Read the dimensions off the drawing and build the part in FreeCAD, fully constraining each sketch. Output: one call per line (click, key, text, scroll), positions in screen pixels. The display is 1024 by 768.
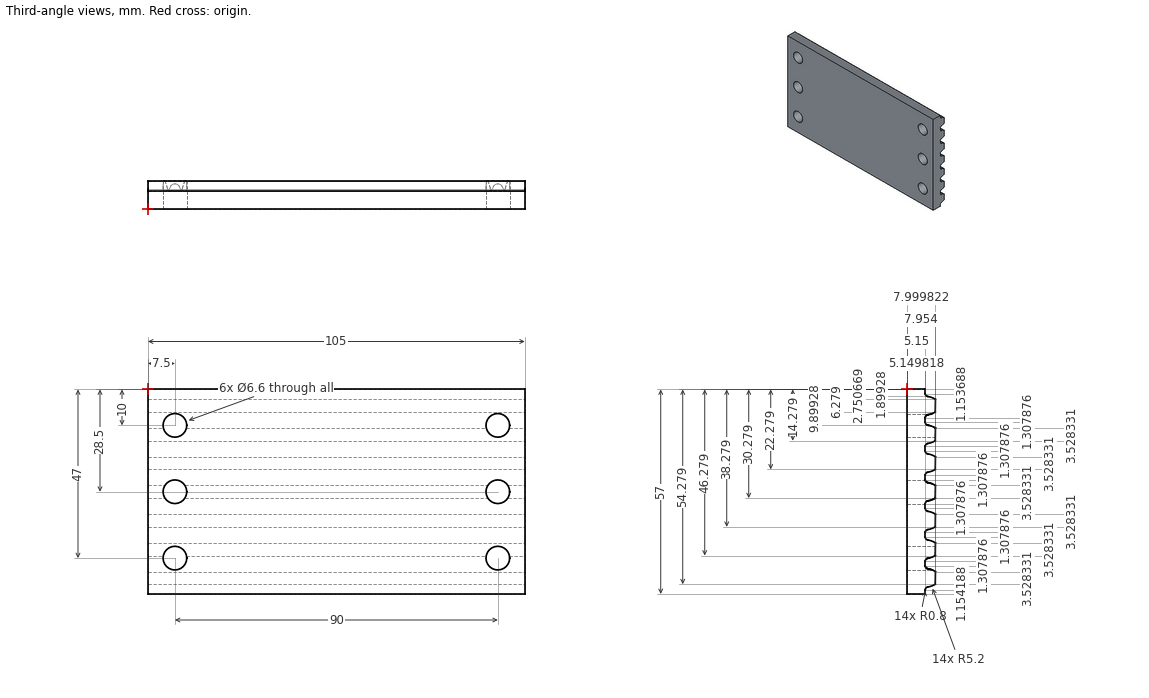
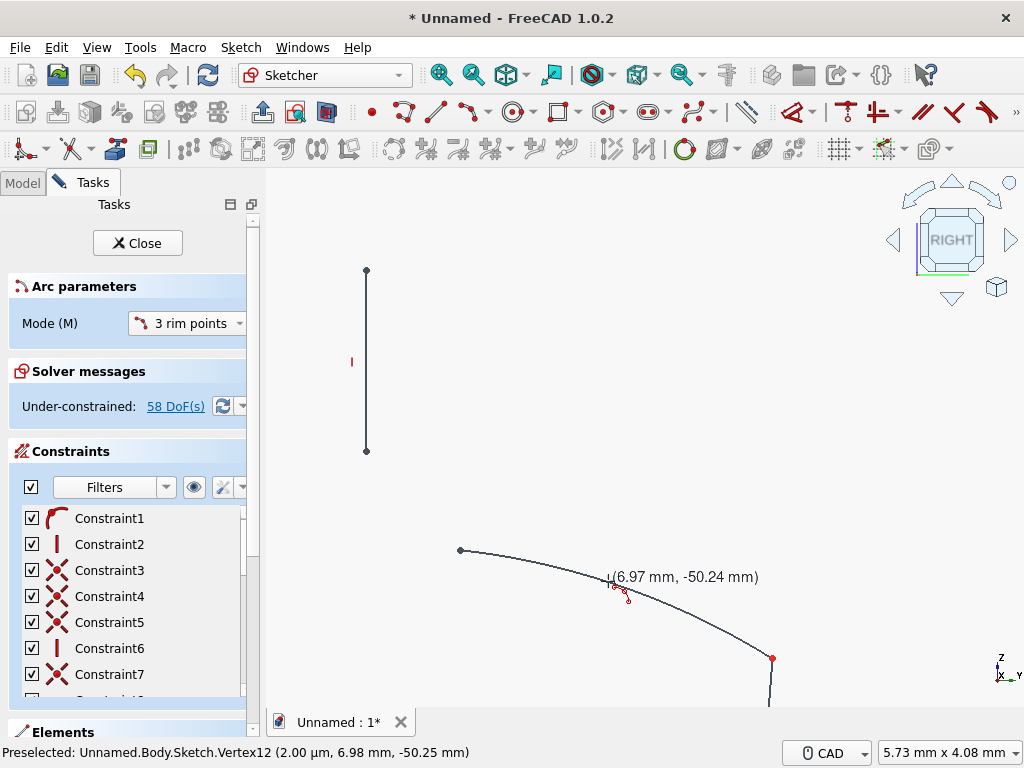
scroll(595, 581, down, 15)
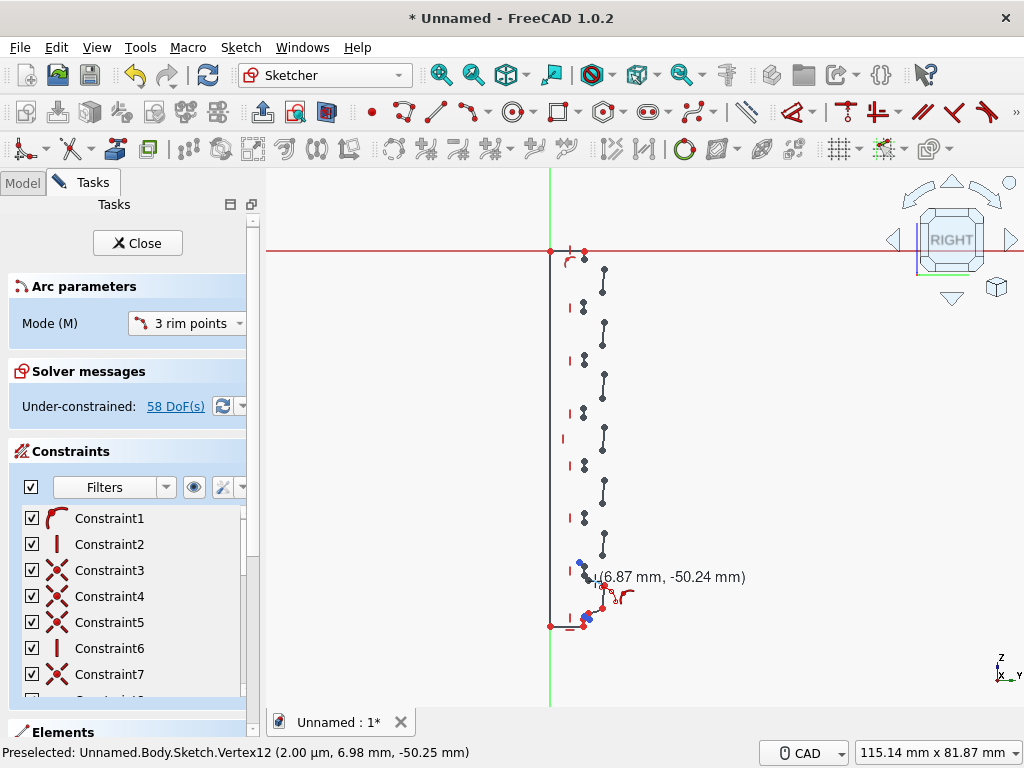
scroll(589, 580, up, 7)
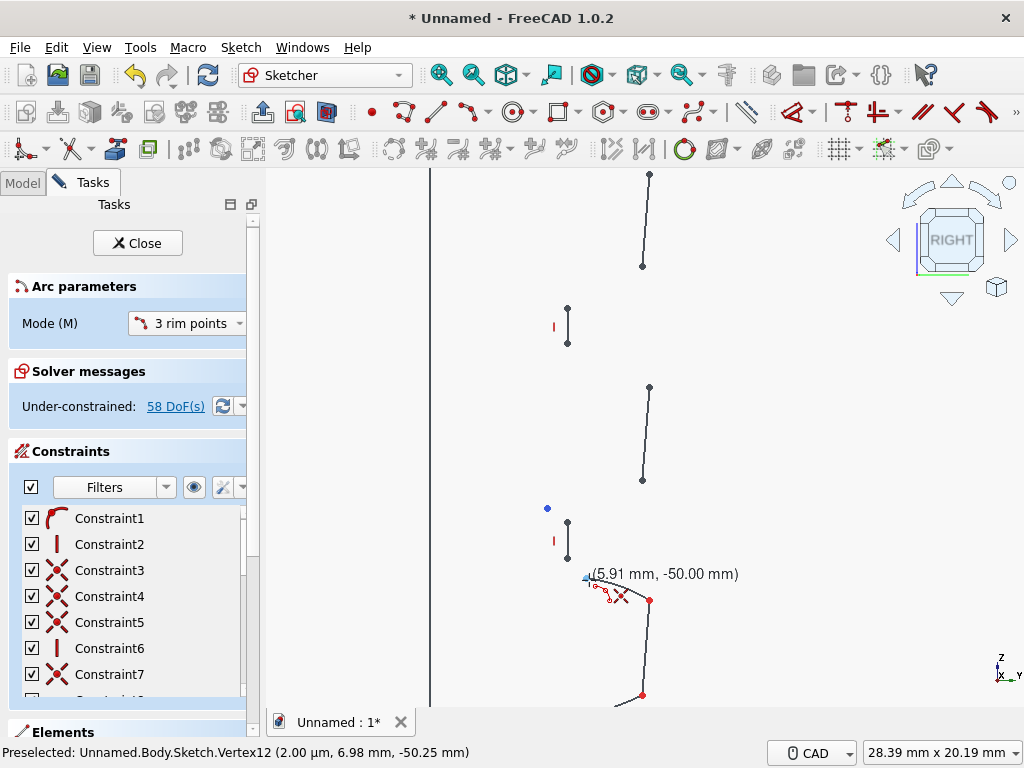
click(587, 578)
click(568, 558)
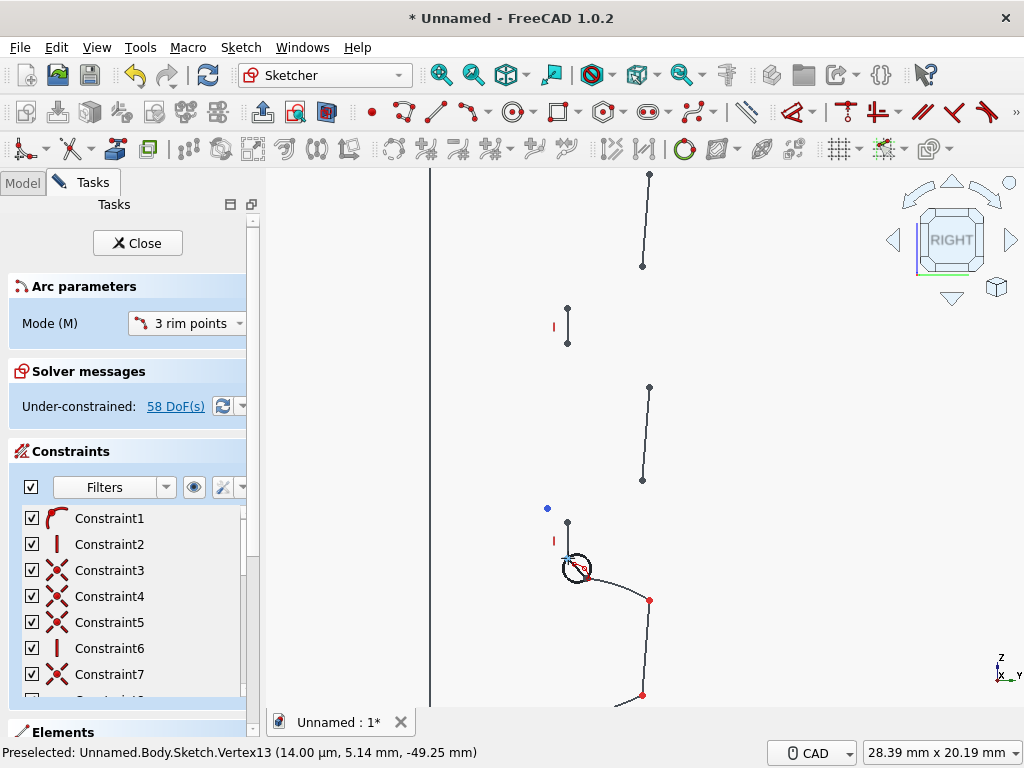
scroll(573, 570, up, 6)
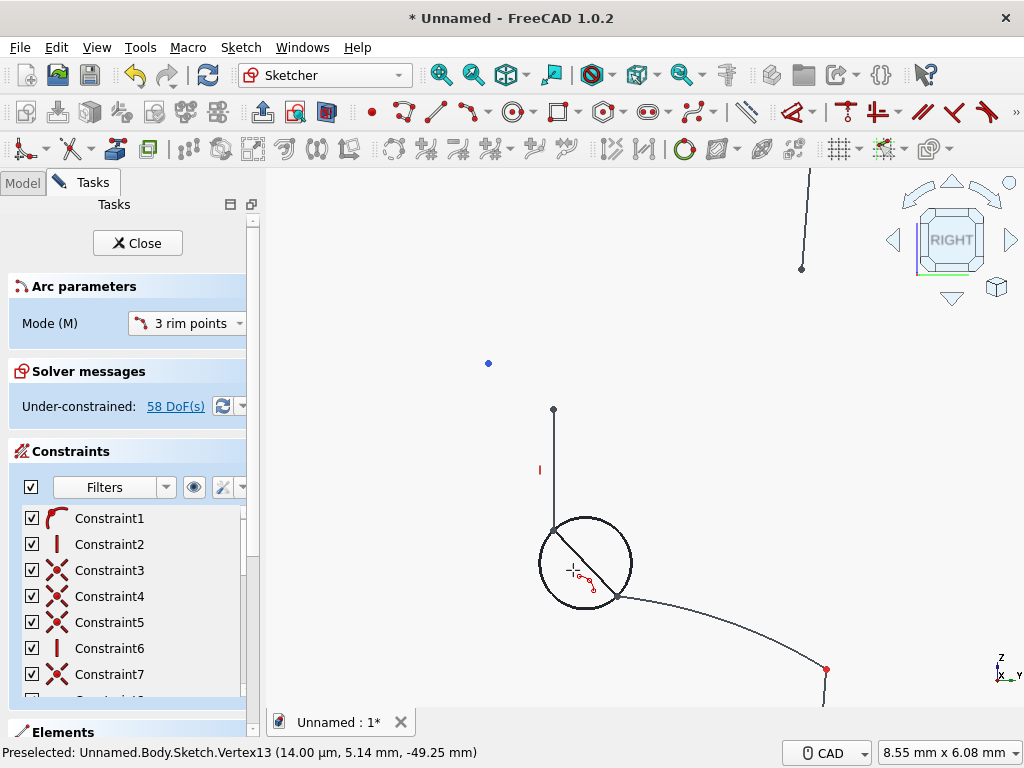
click(572, 568)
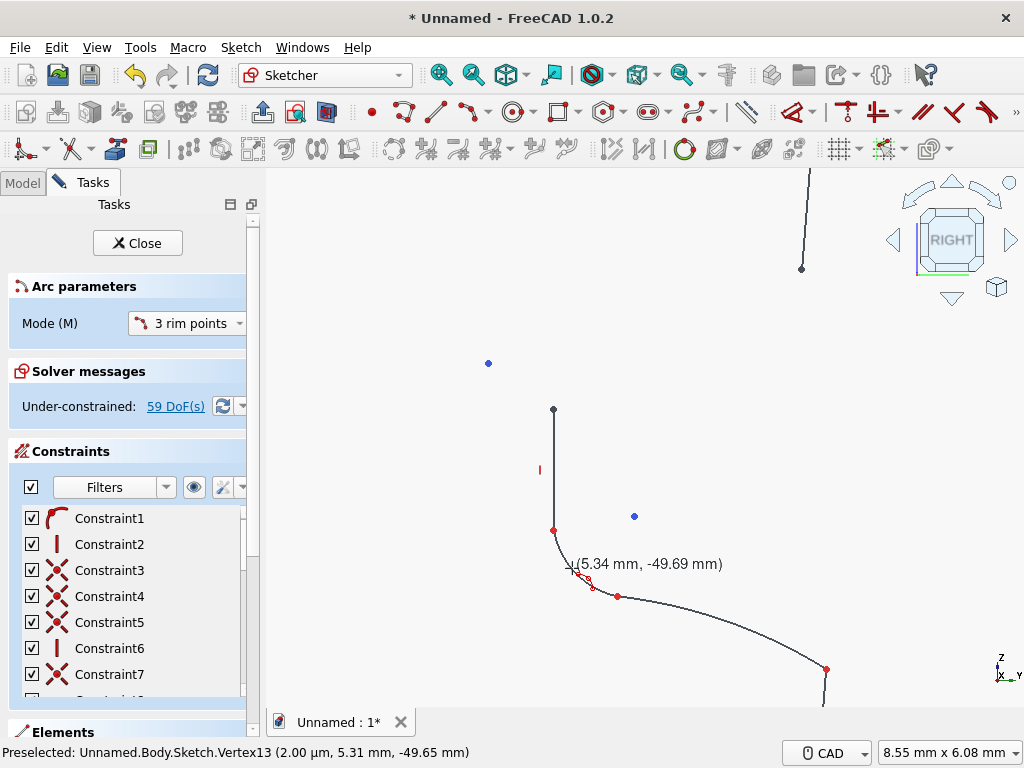
scroll(586, 578, down, 13)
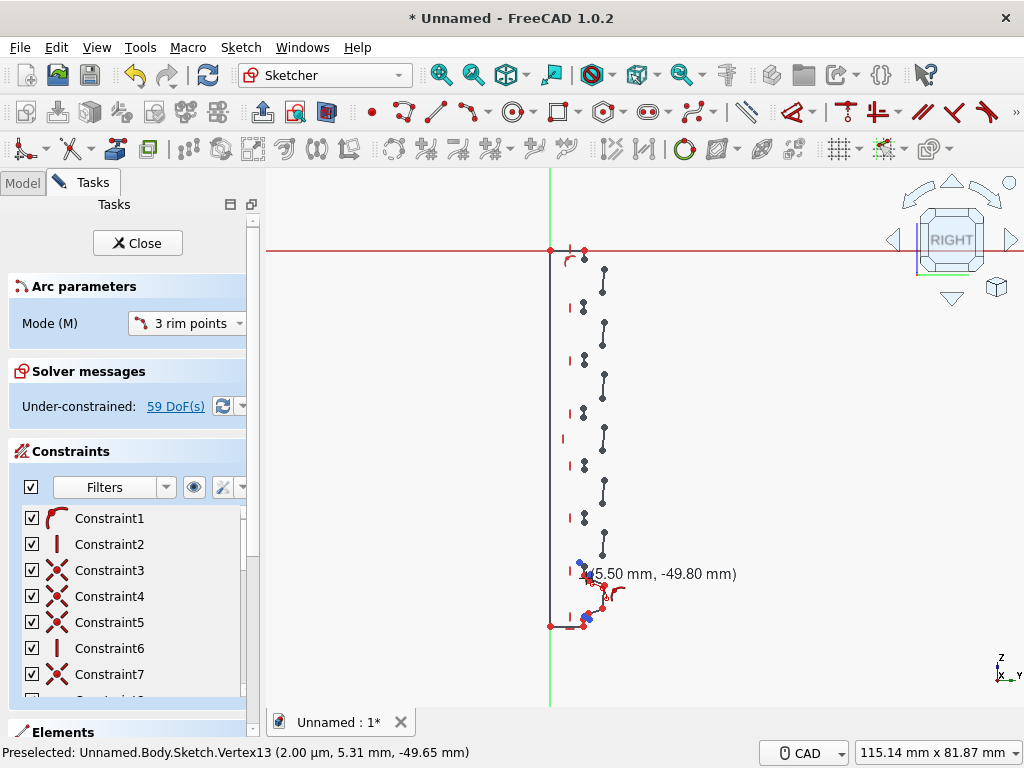
scroll(584, 566, up, 7)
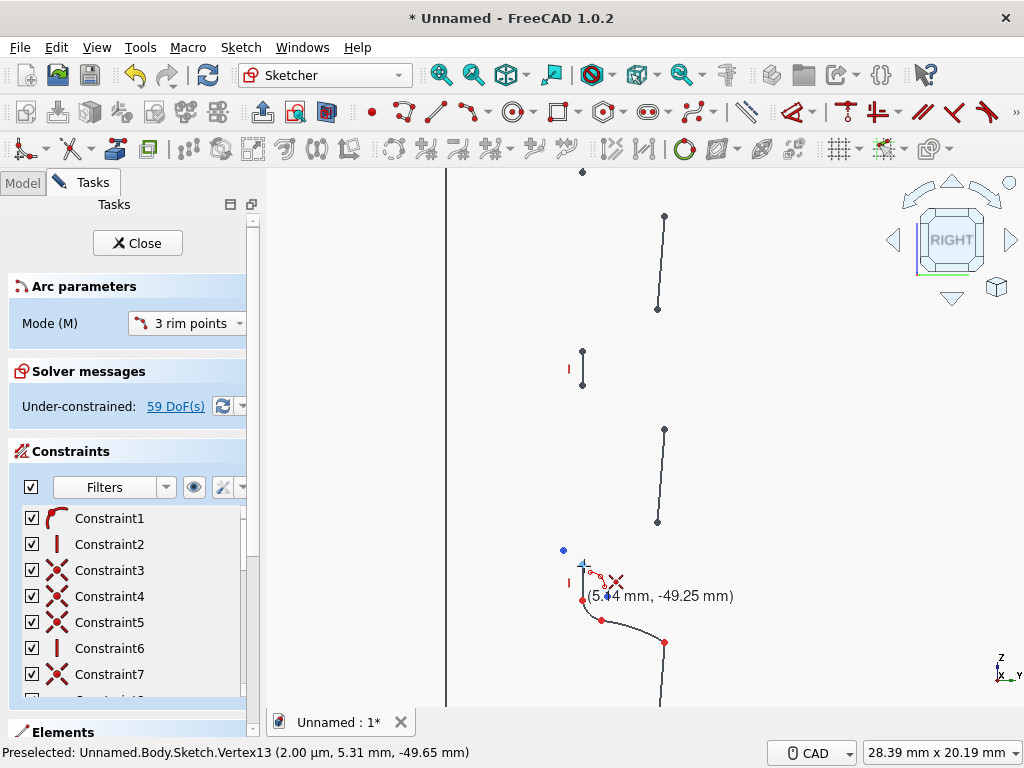
click(583, 564)
click(602, 542)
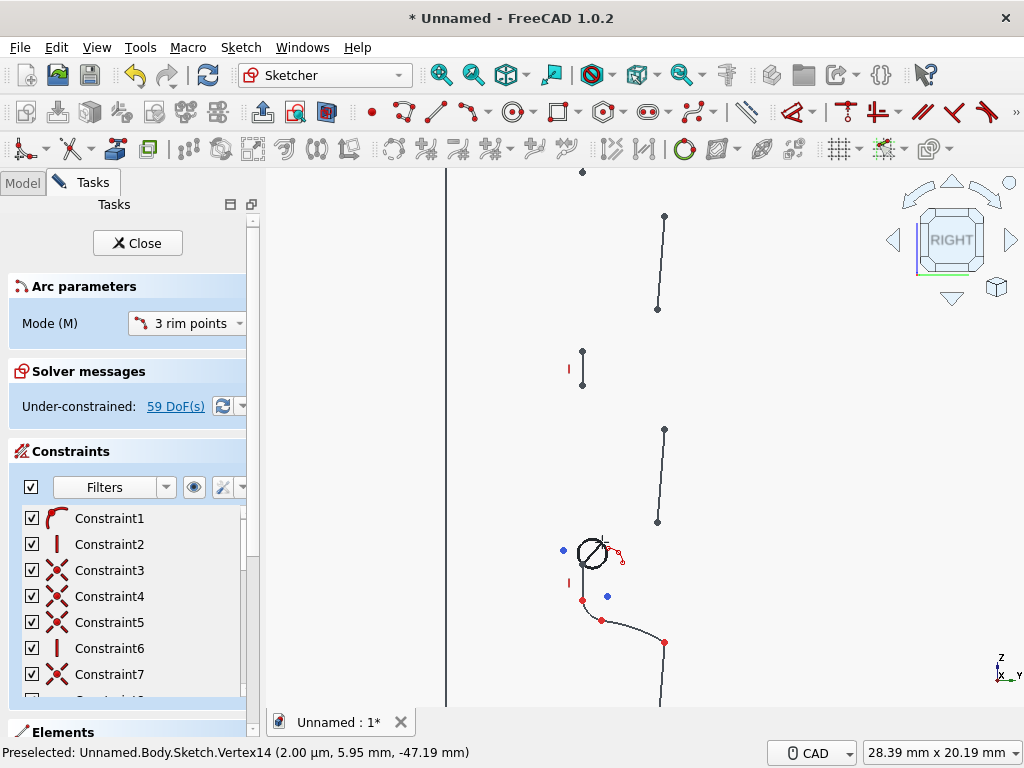
scroll(588, 549, up, 6)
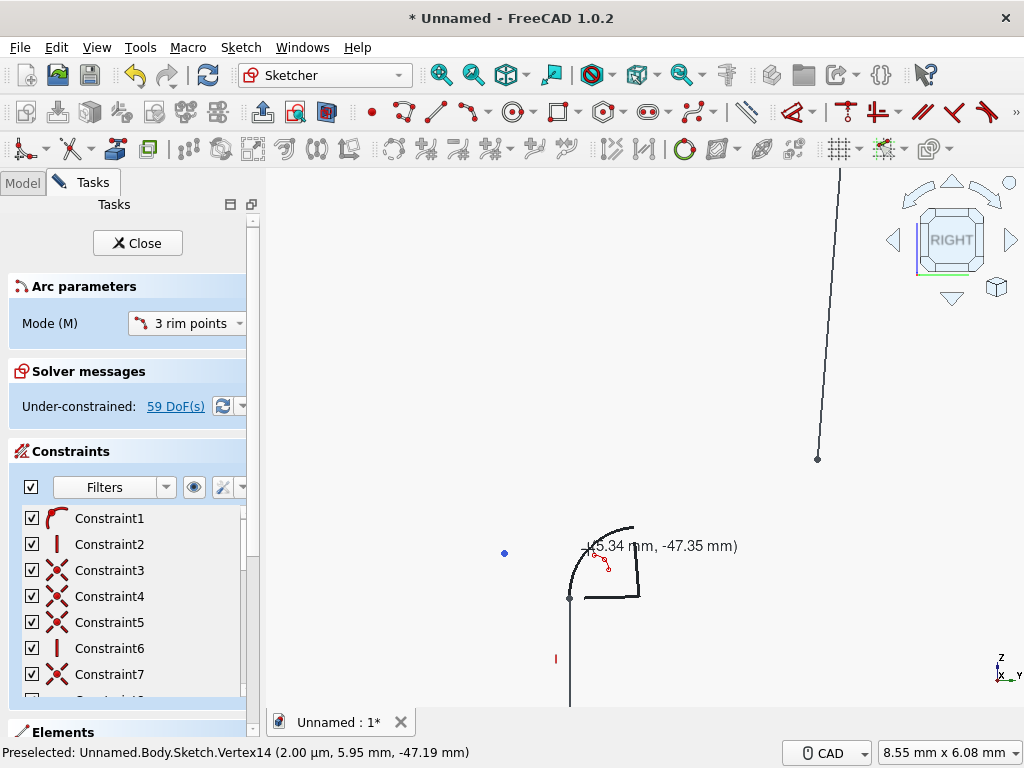
click(588, 548)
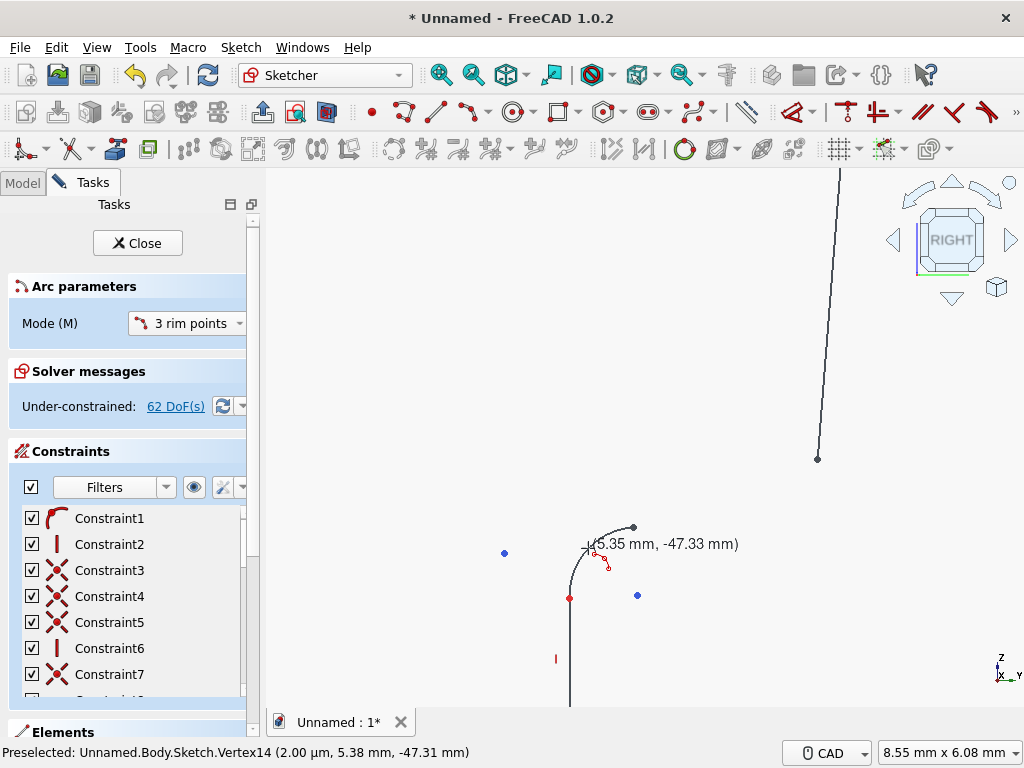
scroll(585, 562, down, 13)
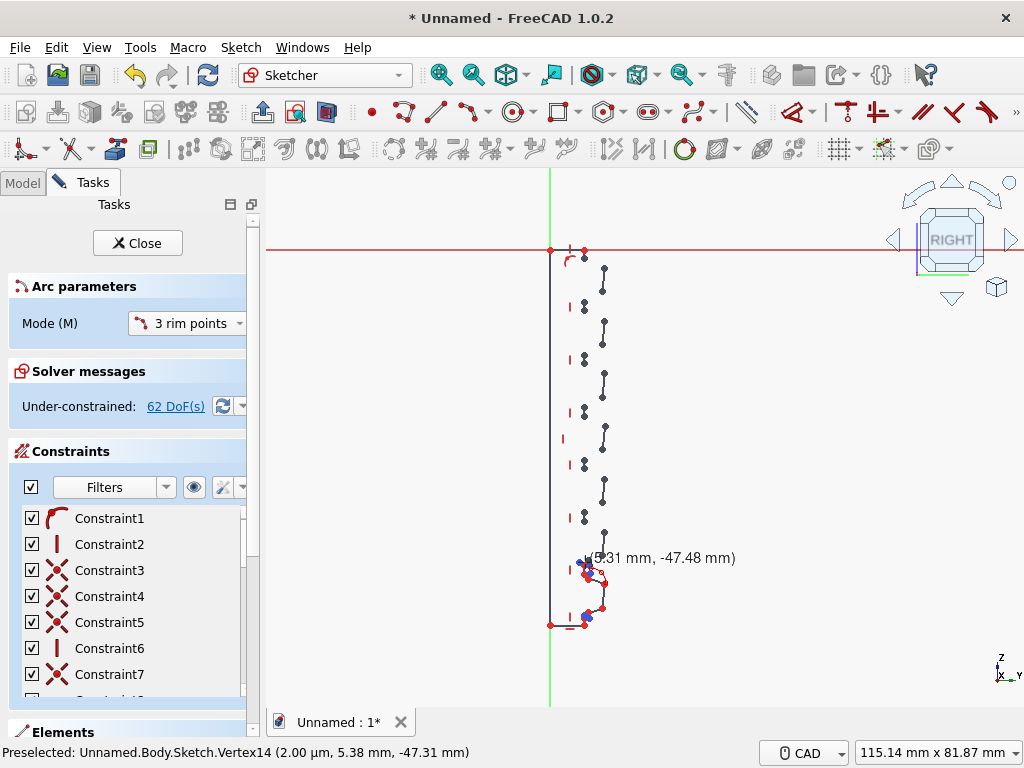
scroll(589, 560, up, 6)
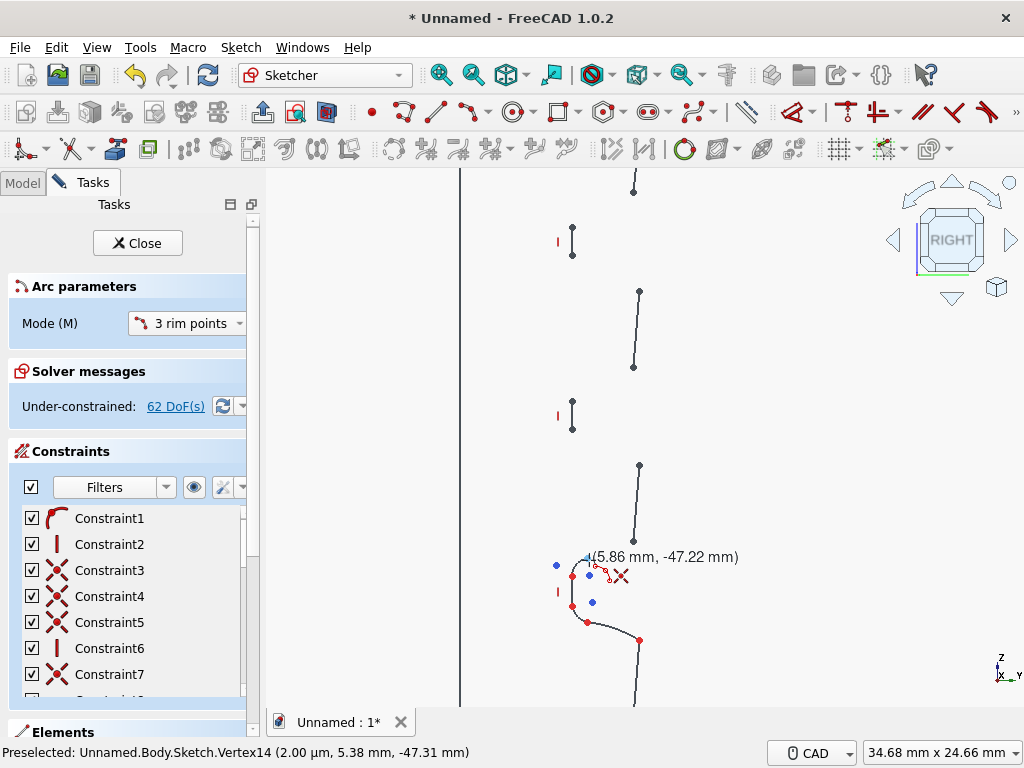
click(588, 559)
click(633, 542)